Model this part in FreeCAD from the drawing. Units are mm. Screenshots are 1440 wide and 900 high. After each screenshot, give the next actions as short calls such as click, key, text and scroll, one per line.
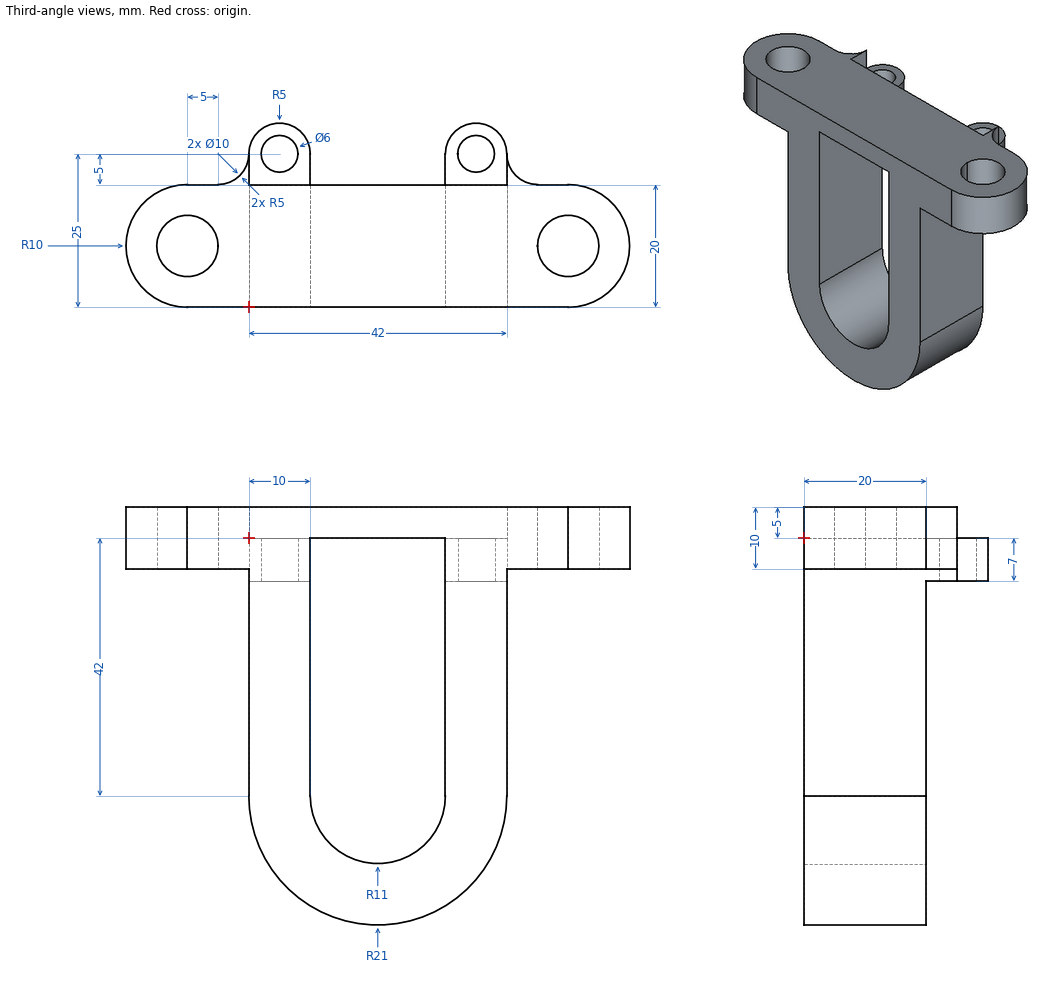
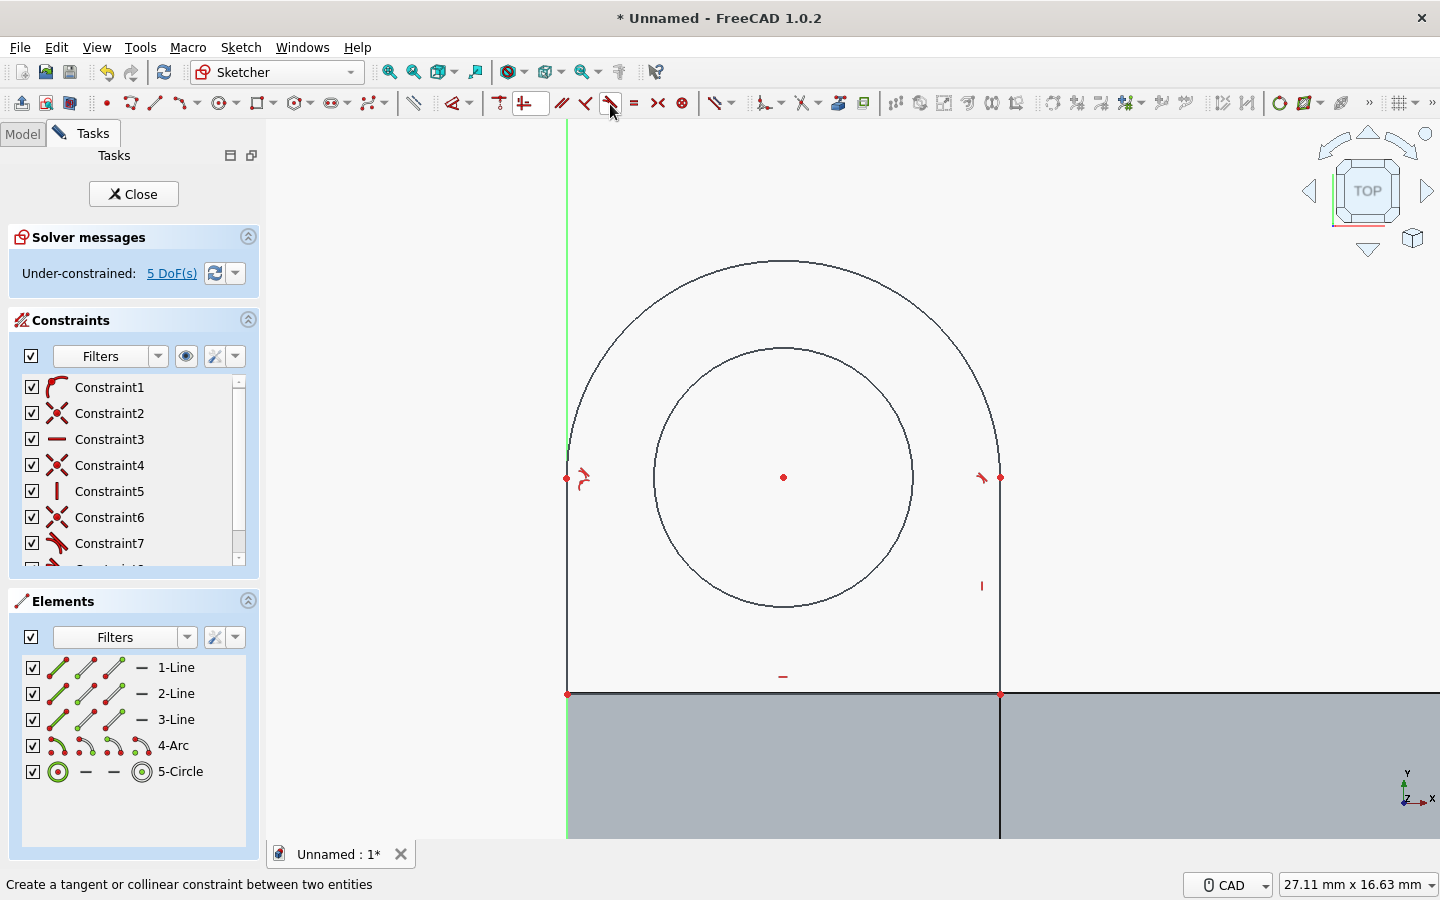
click(567, 543)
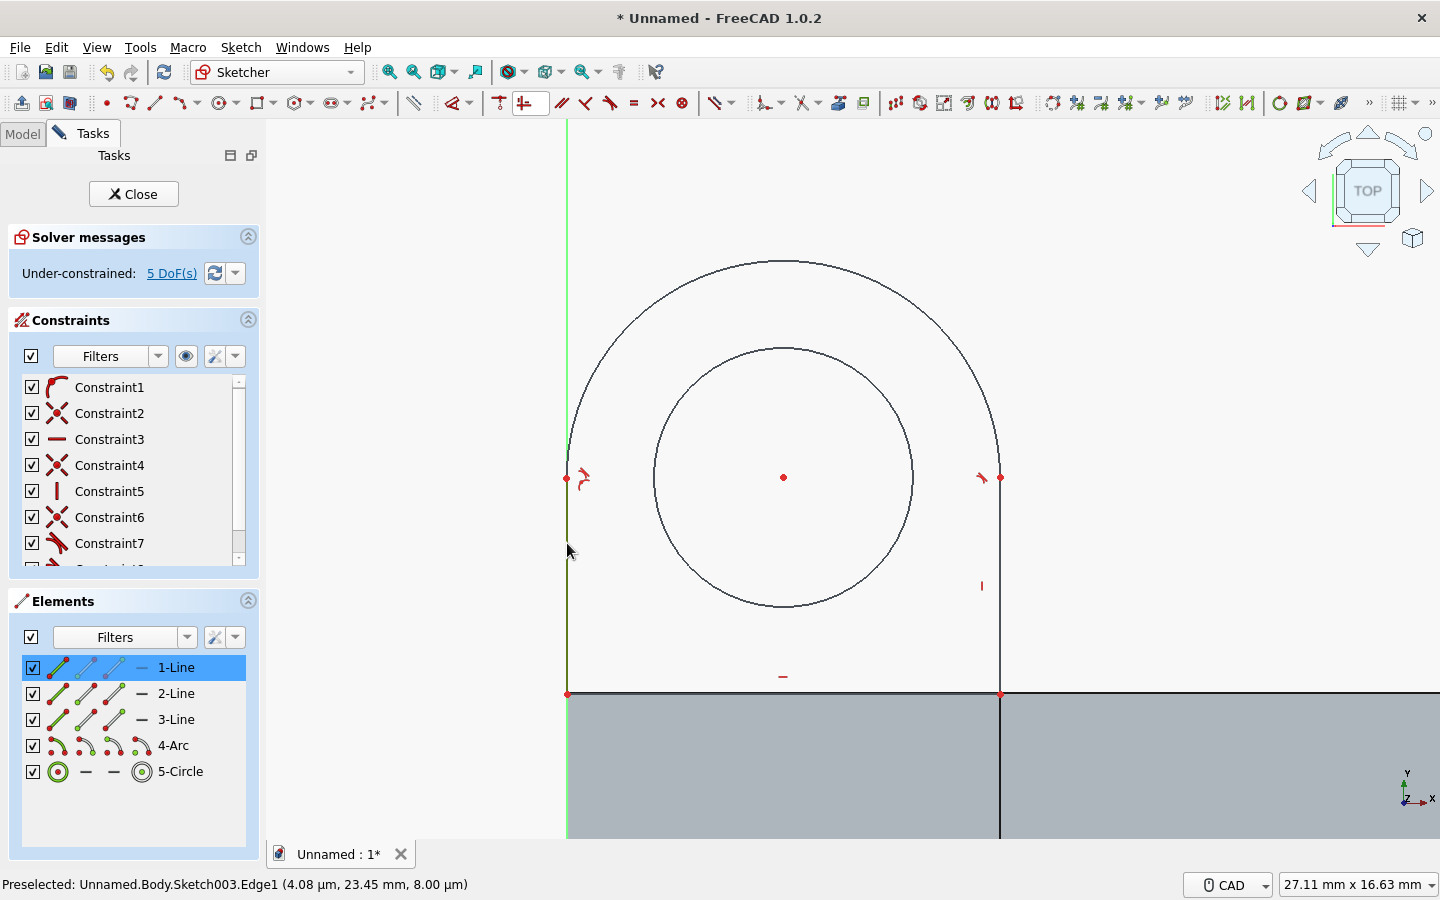
key(v)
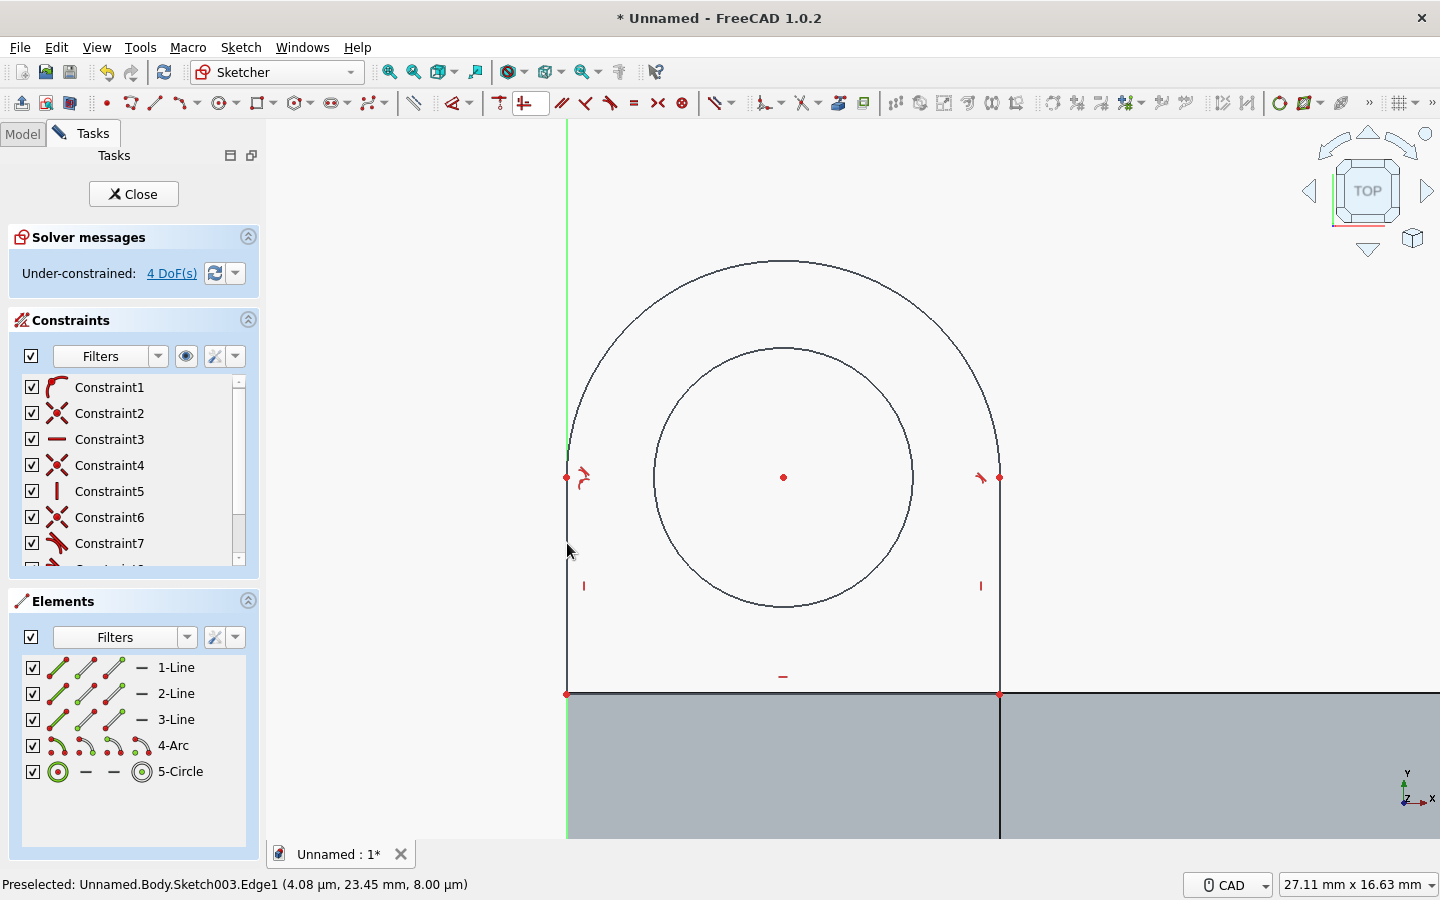
click(452, 104)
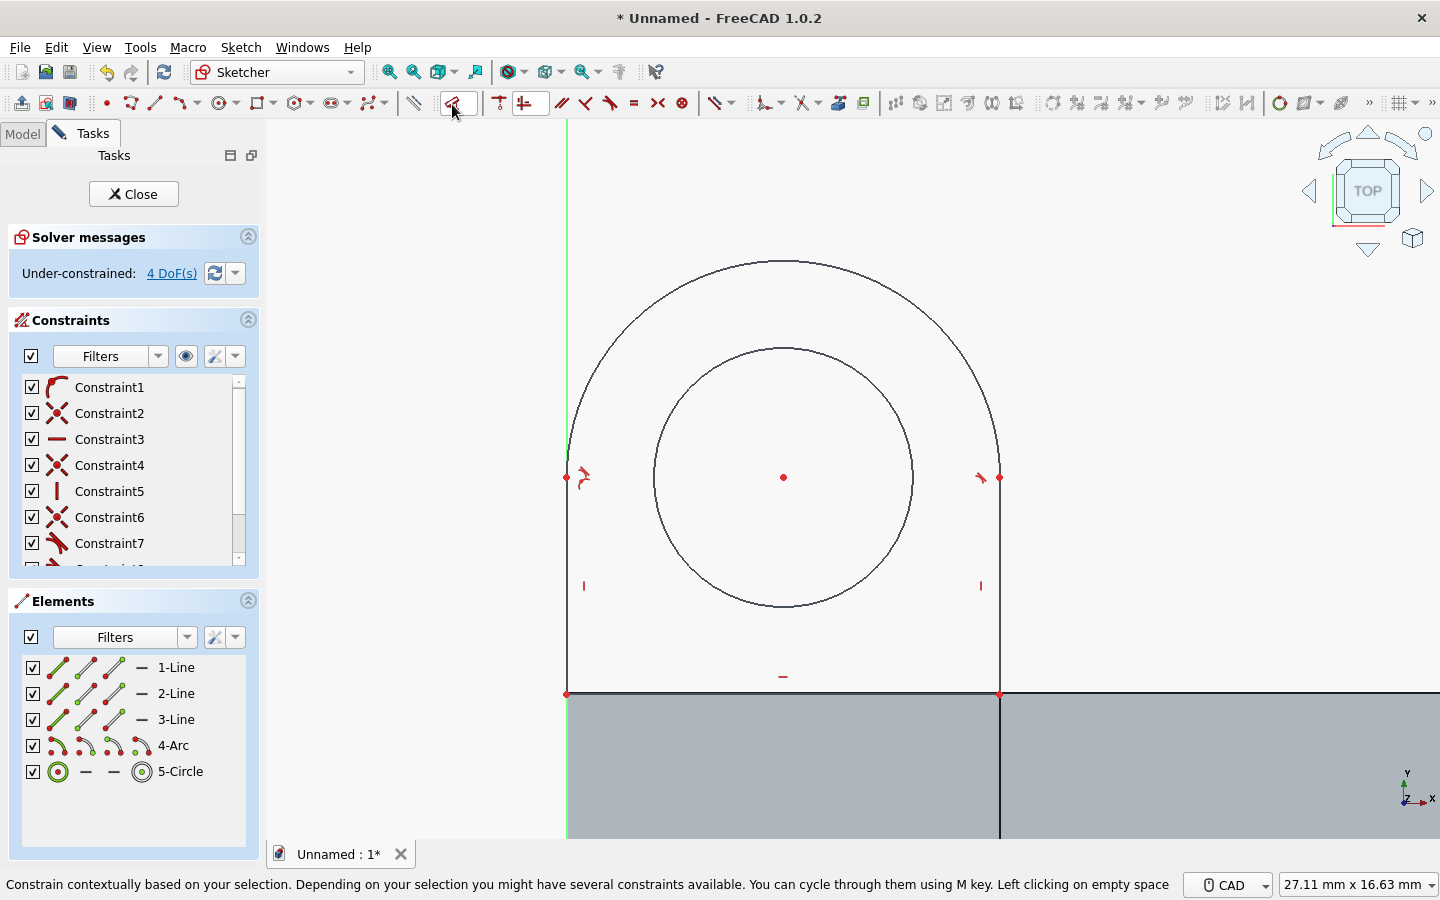
click(911, 302)
click(930, 276)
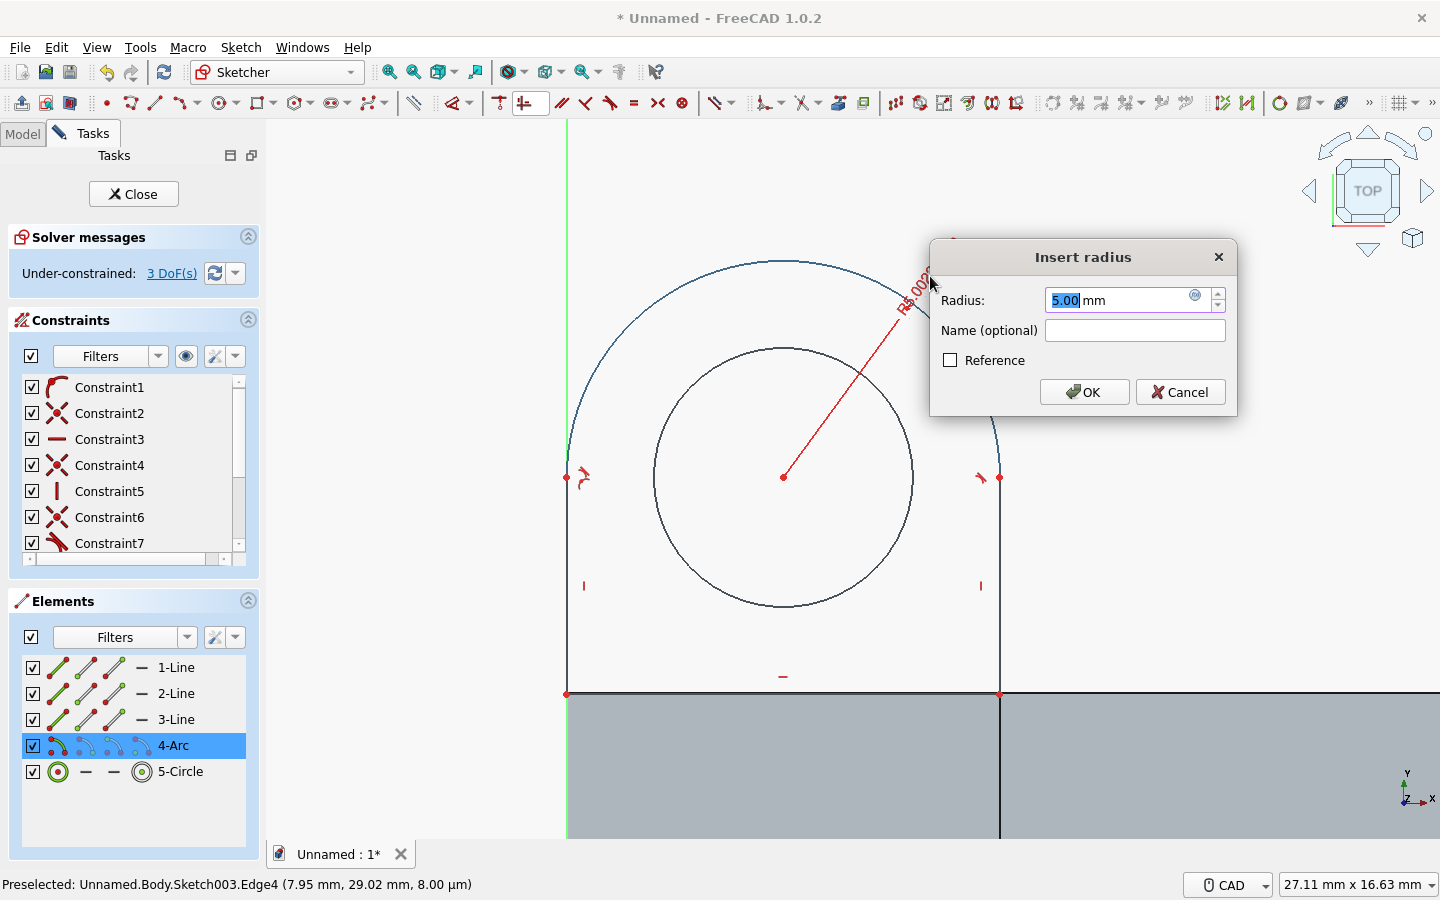
text(5)
key(Return)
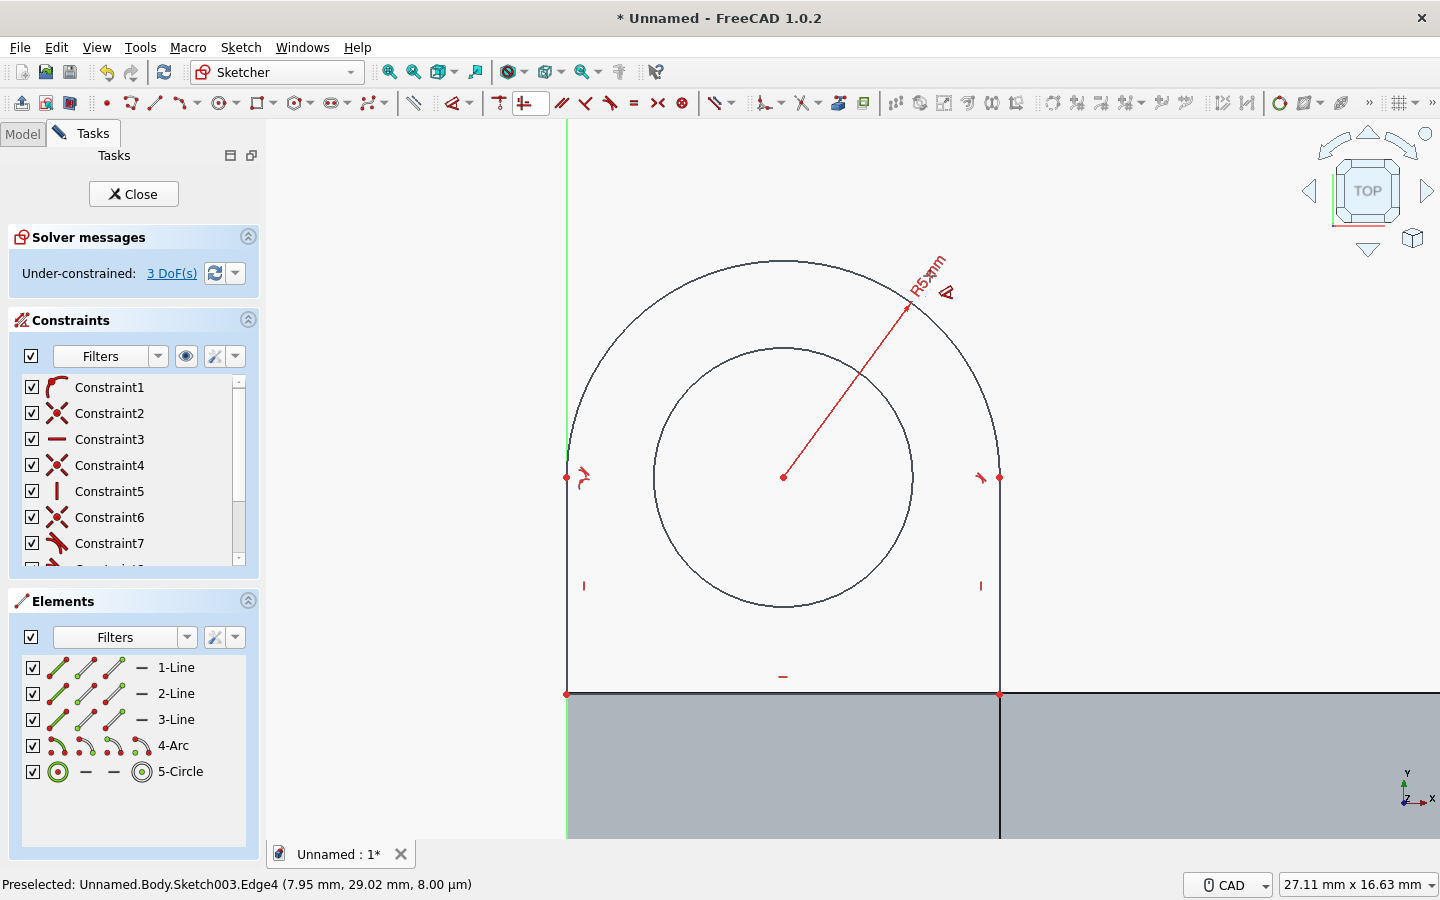
click(875, 386)
click(898, 363)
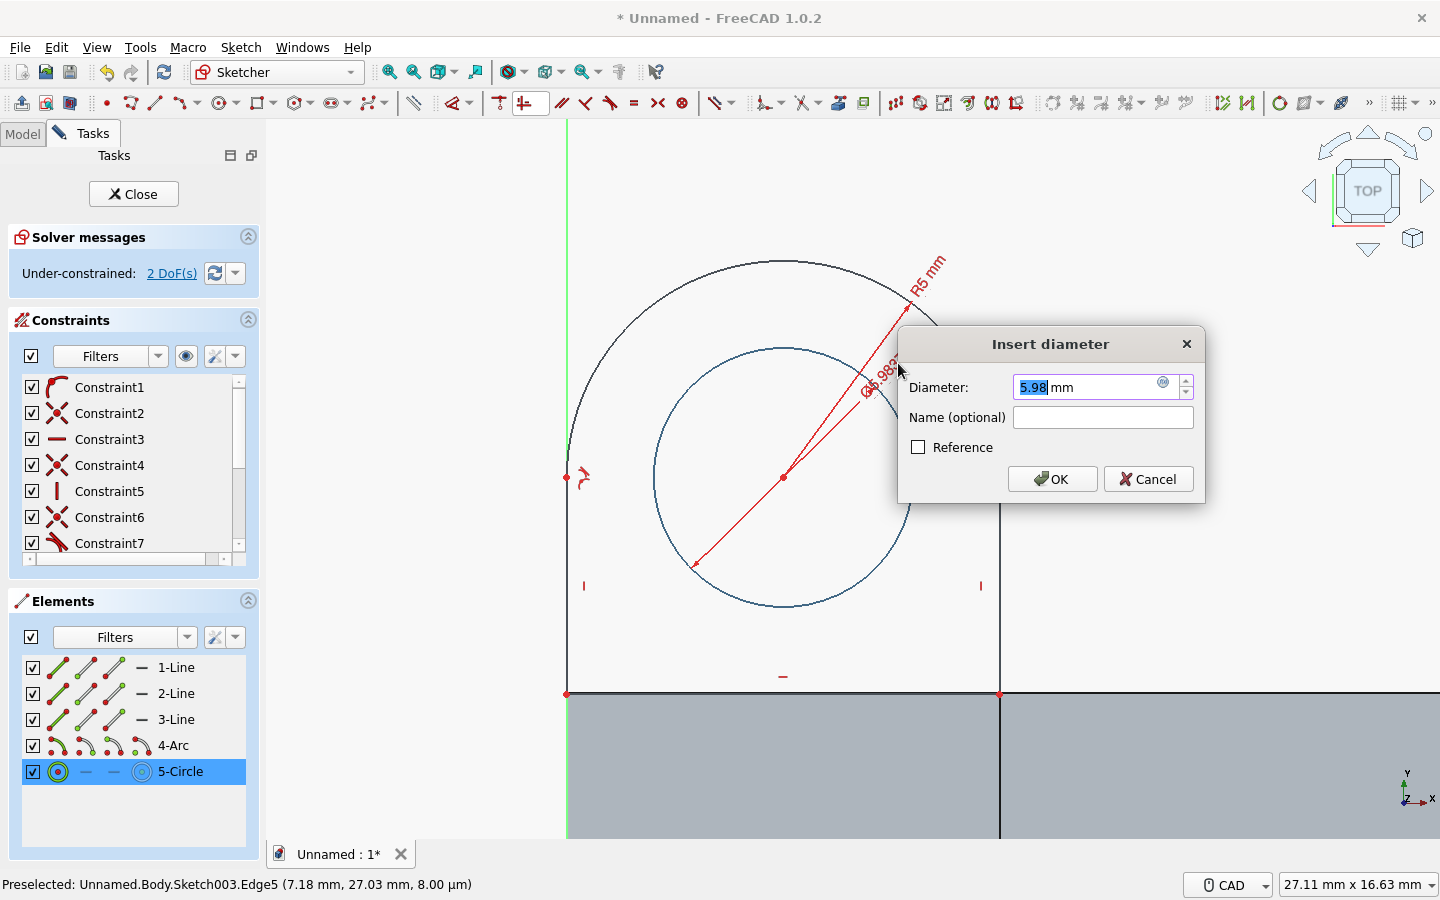
text(6)
key(Return)